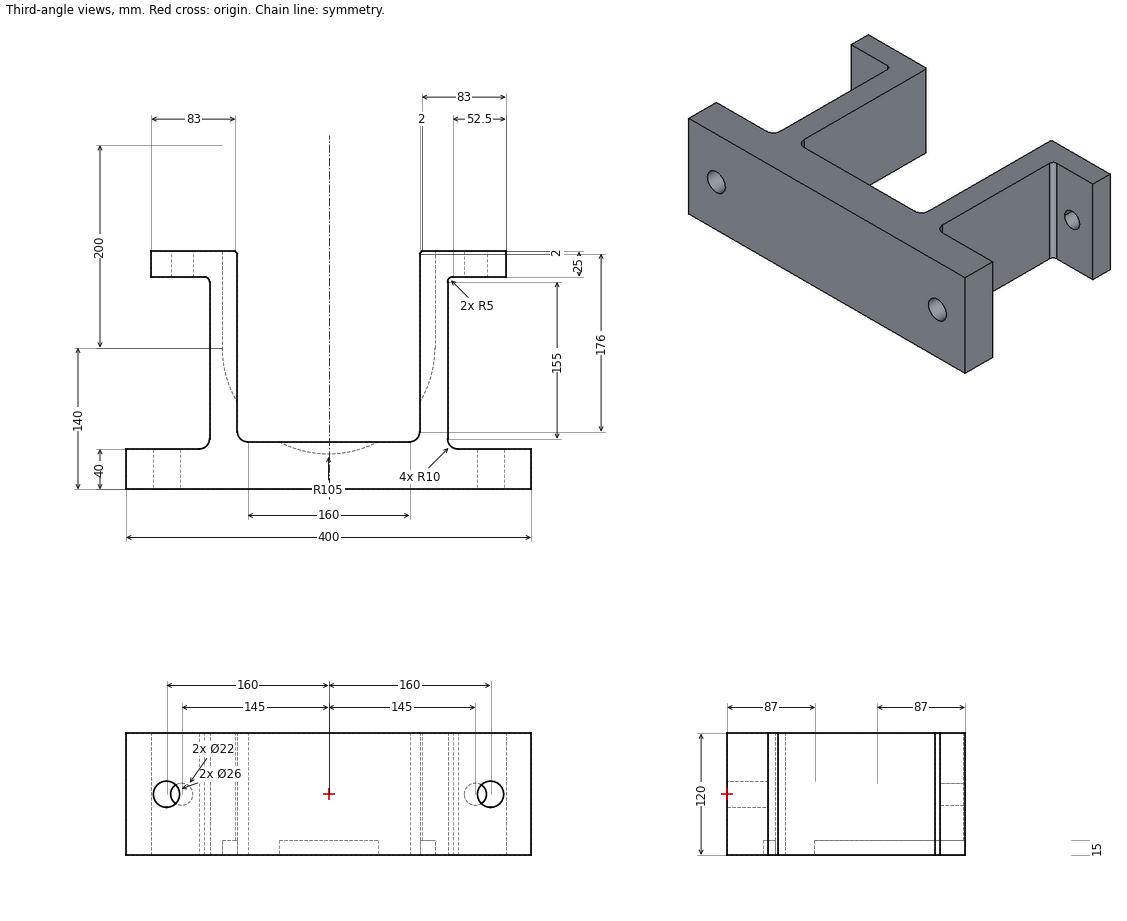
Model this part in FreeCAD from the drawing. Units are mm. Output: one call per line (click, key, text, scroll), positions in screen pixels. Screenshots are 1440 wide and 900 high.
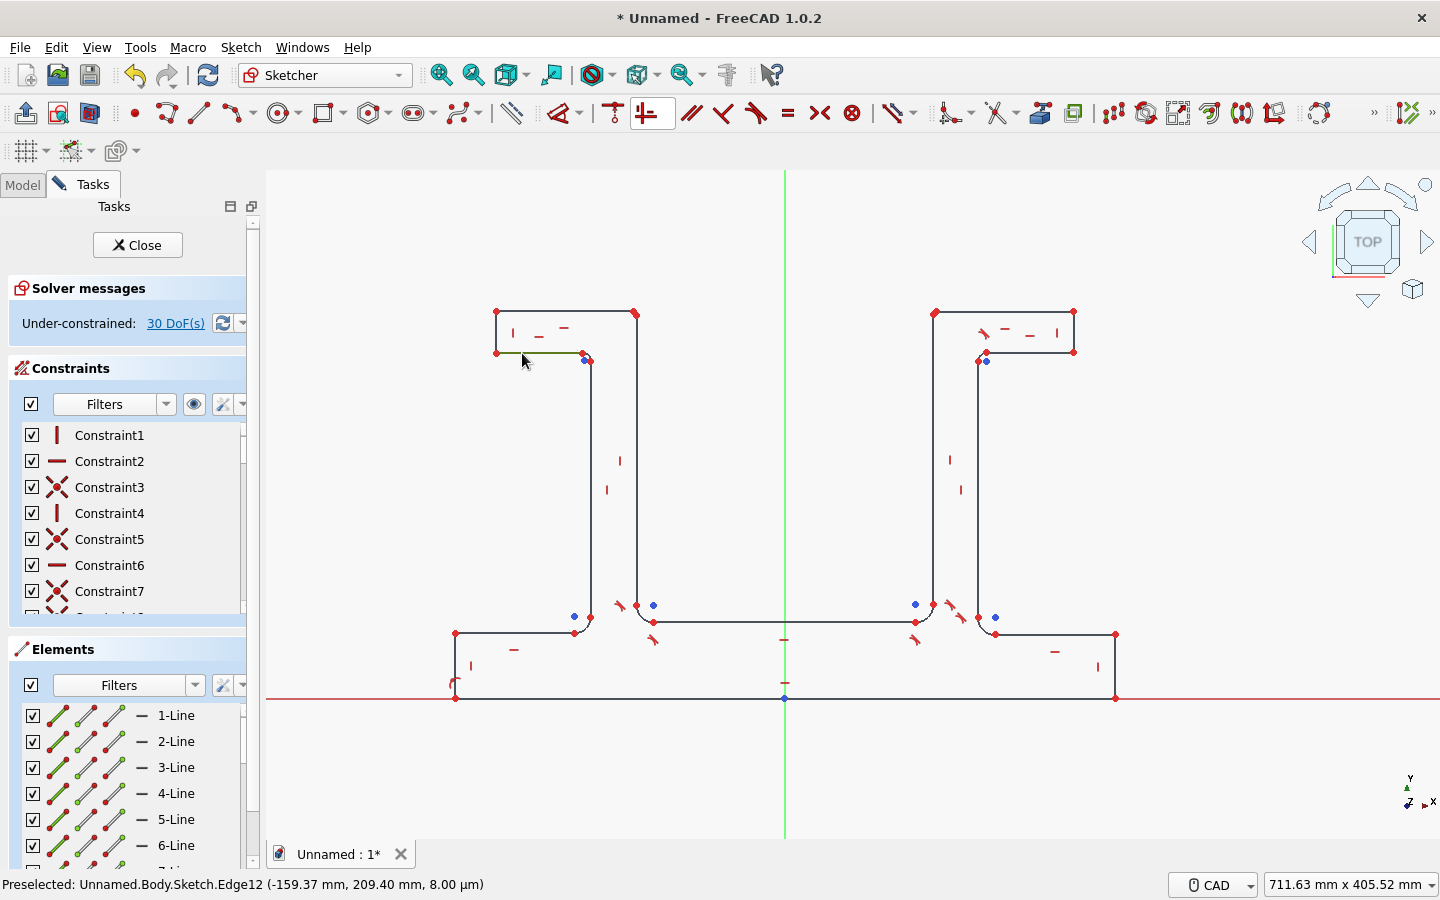
scroll(589, 355, up, 4)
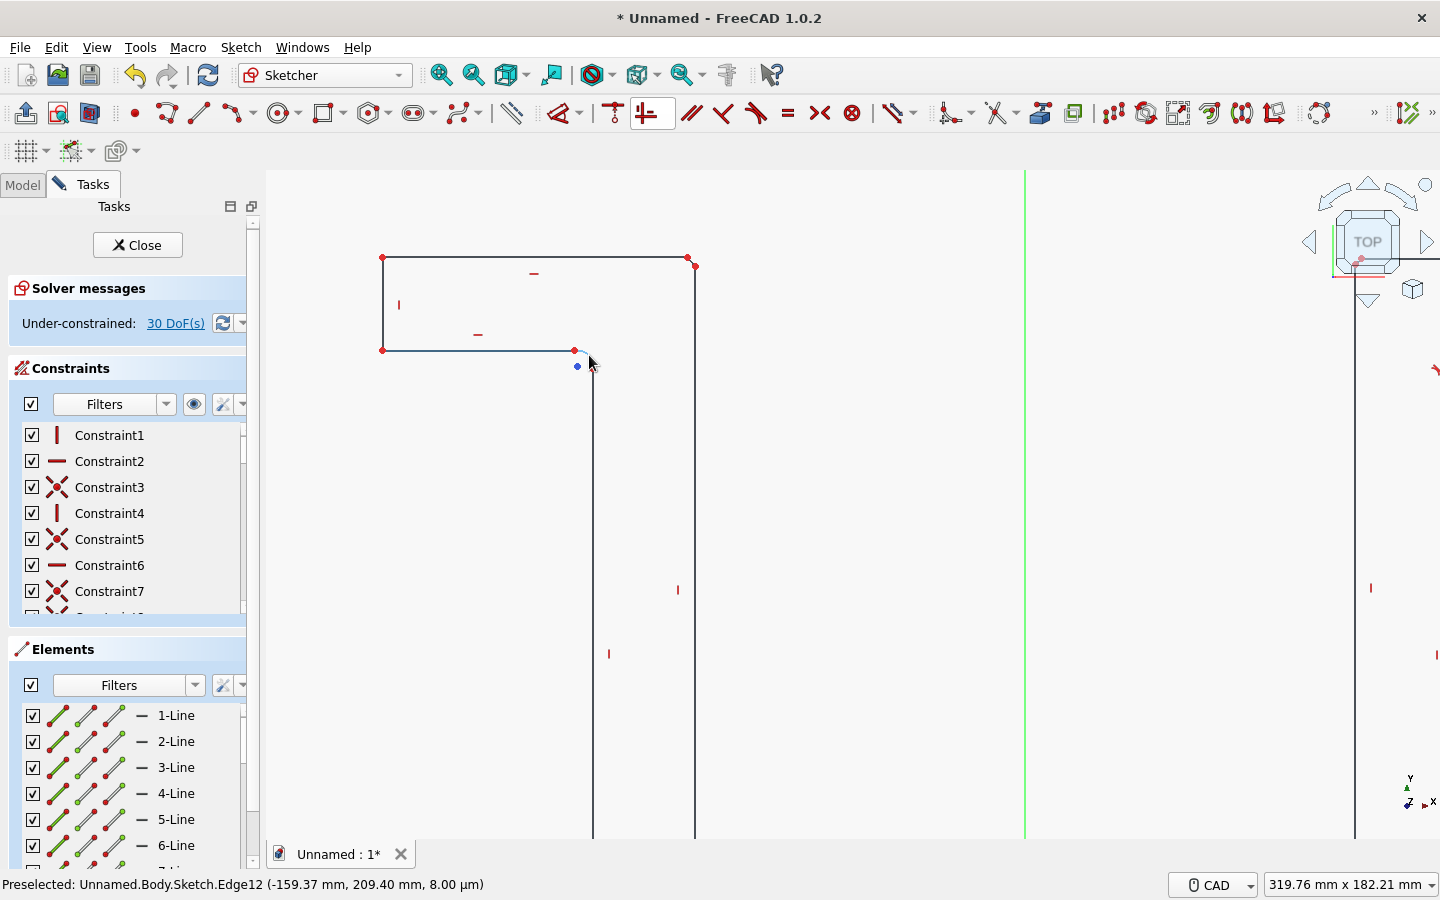
click(588, 355)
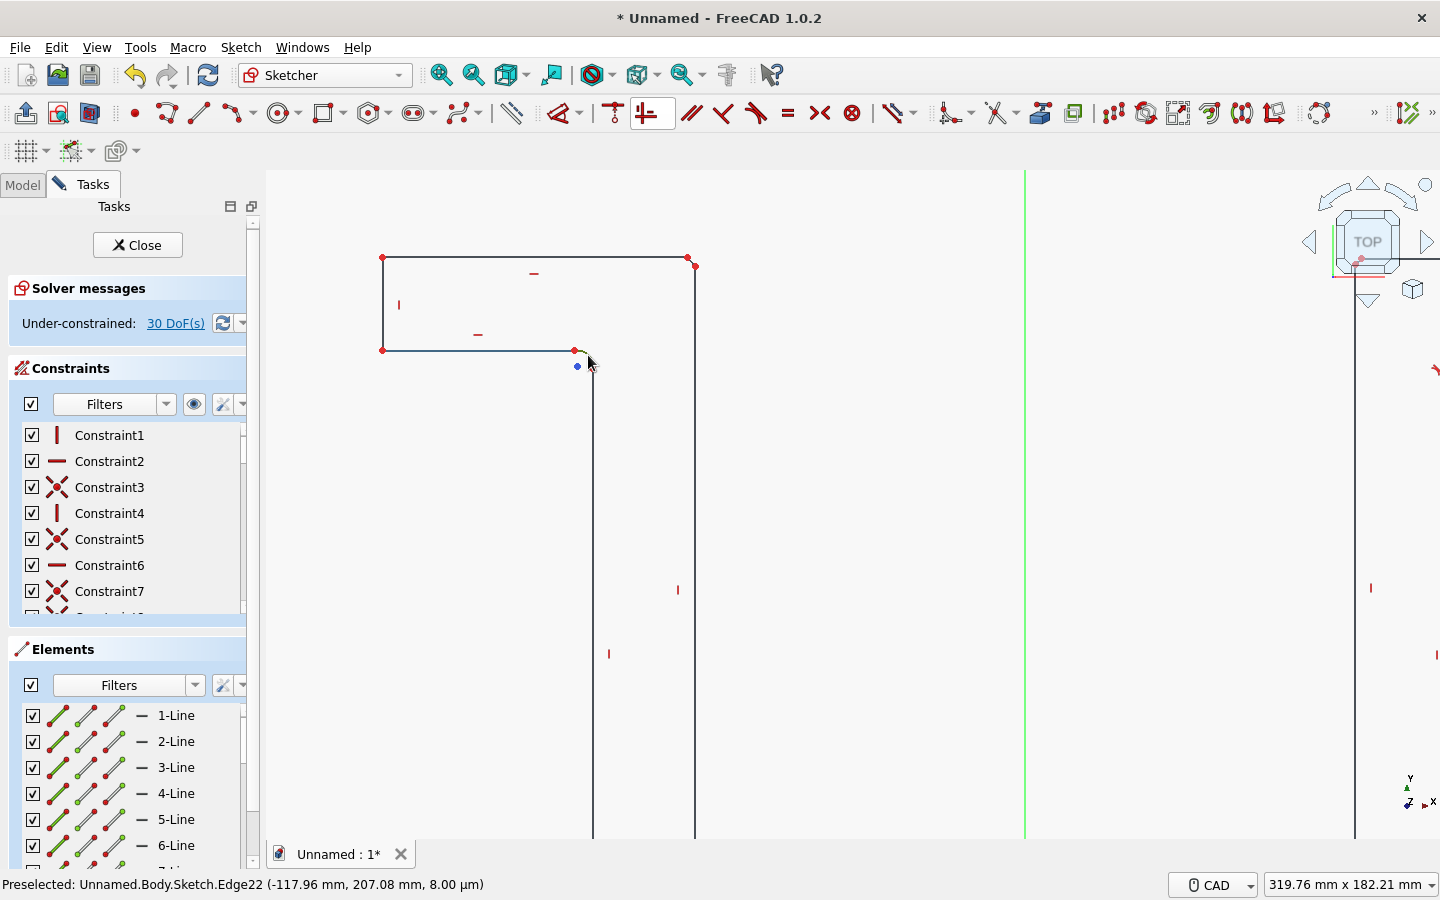
key(t)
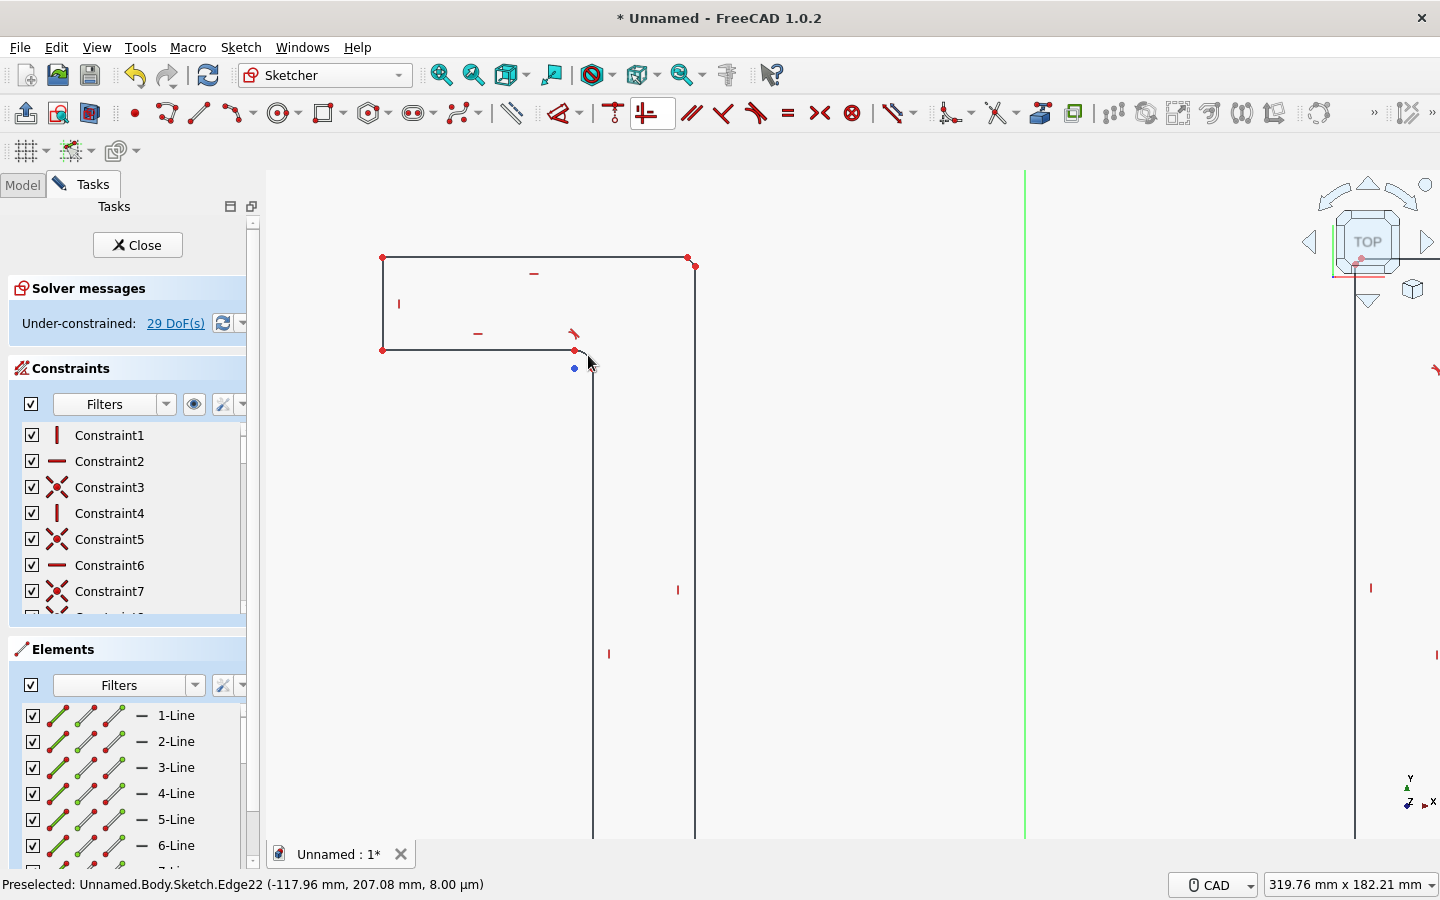
click(593, 539)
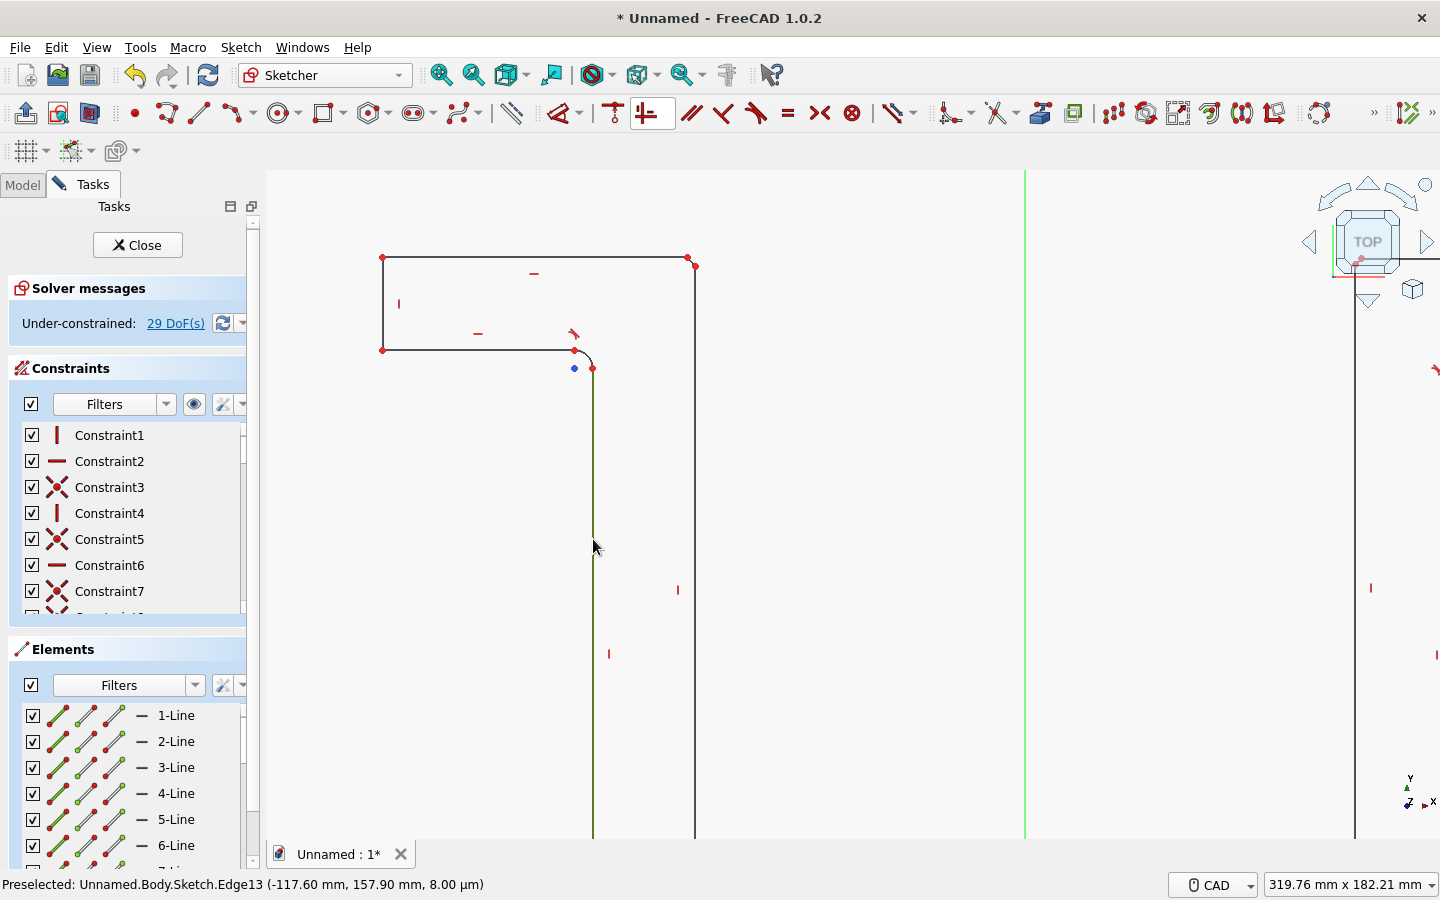
click(587, 355)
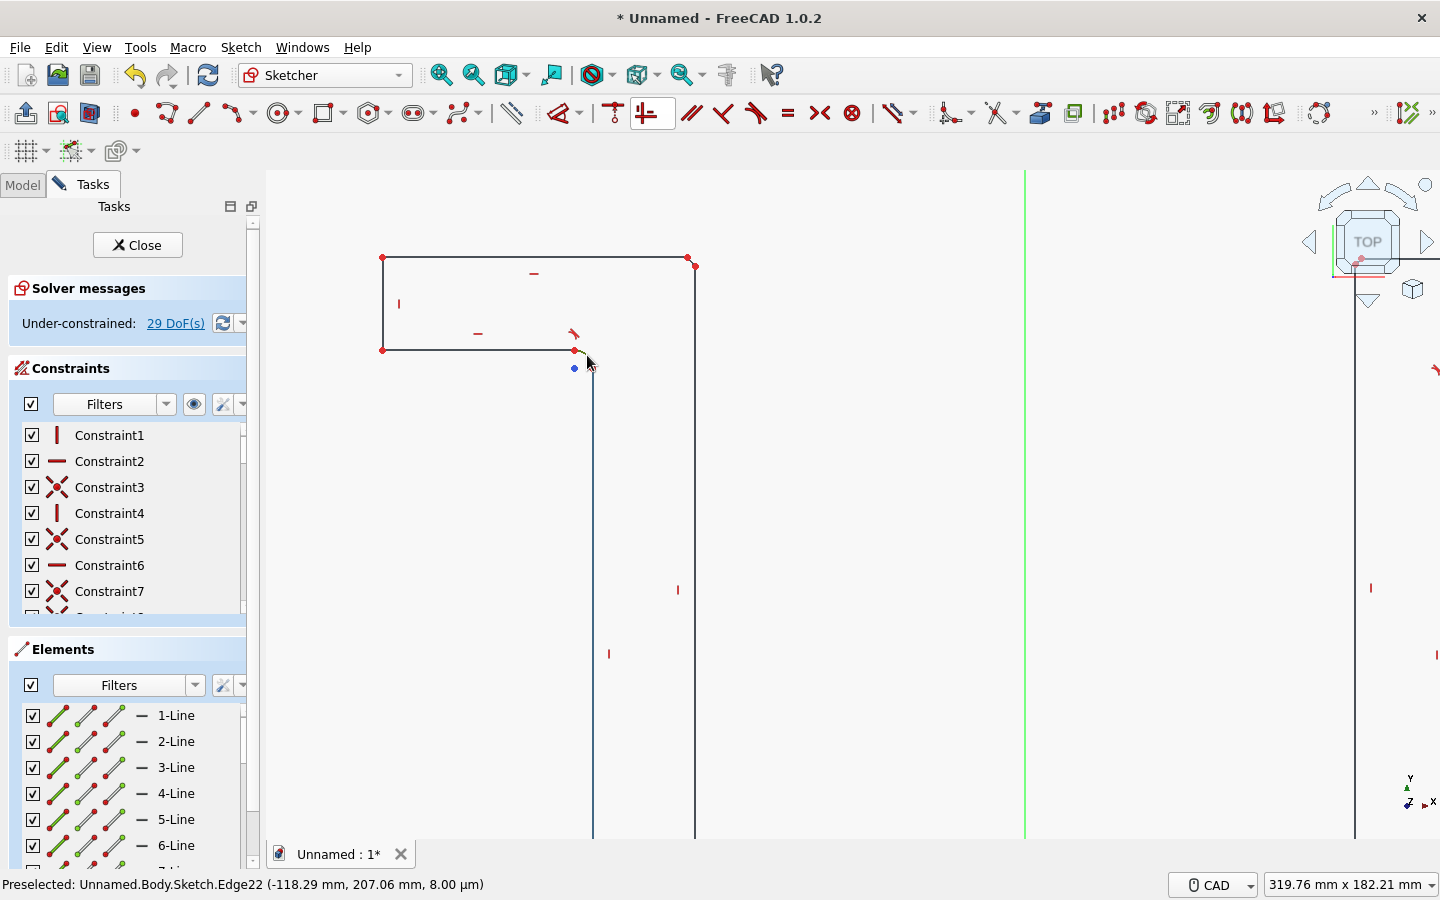
click(756, 114)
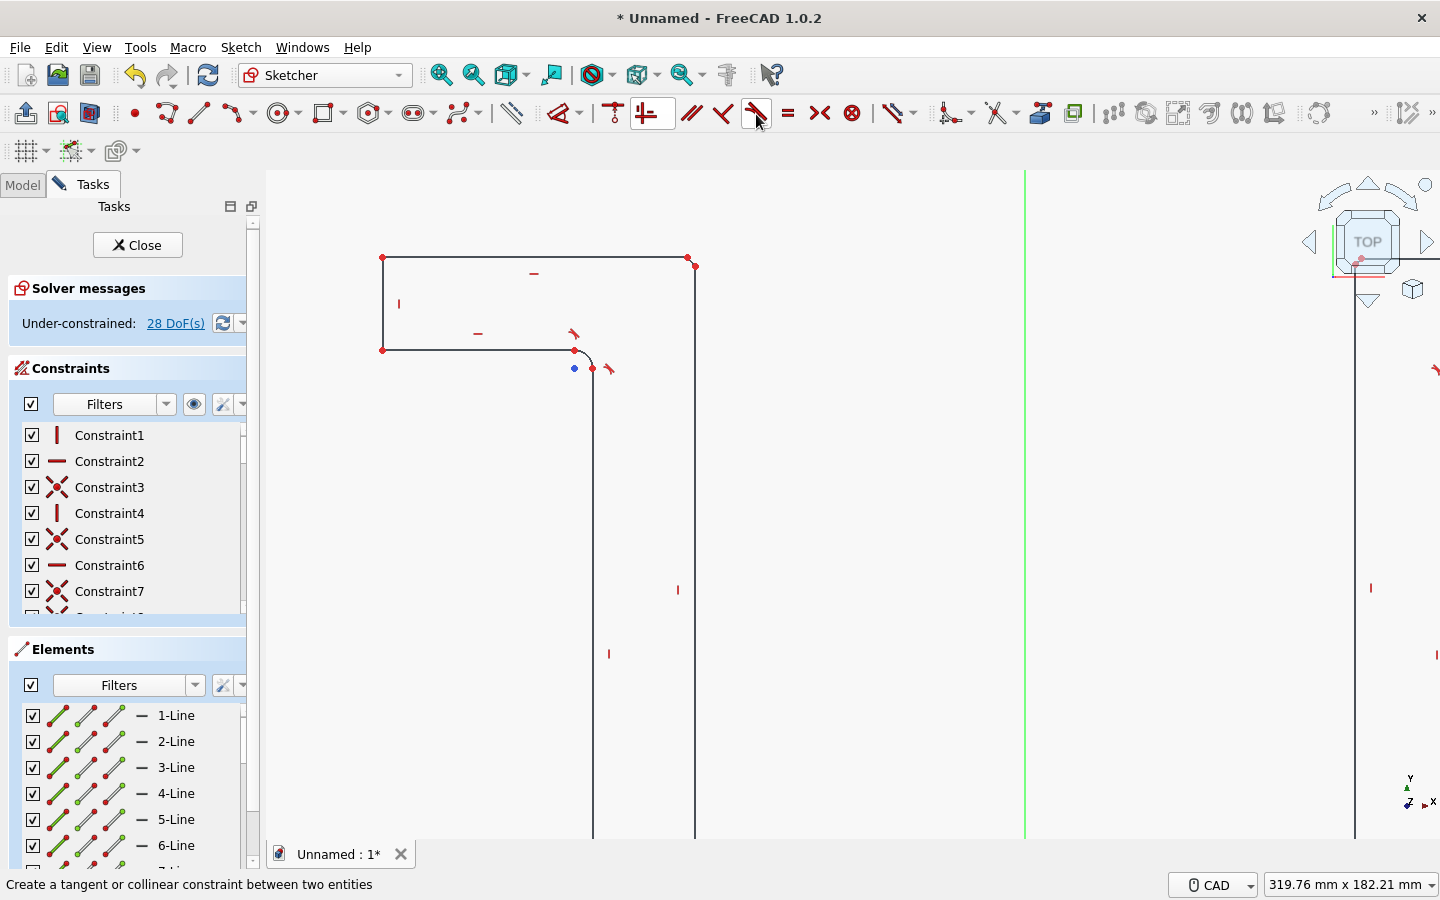
click(593, 540)